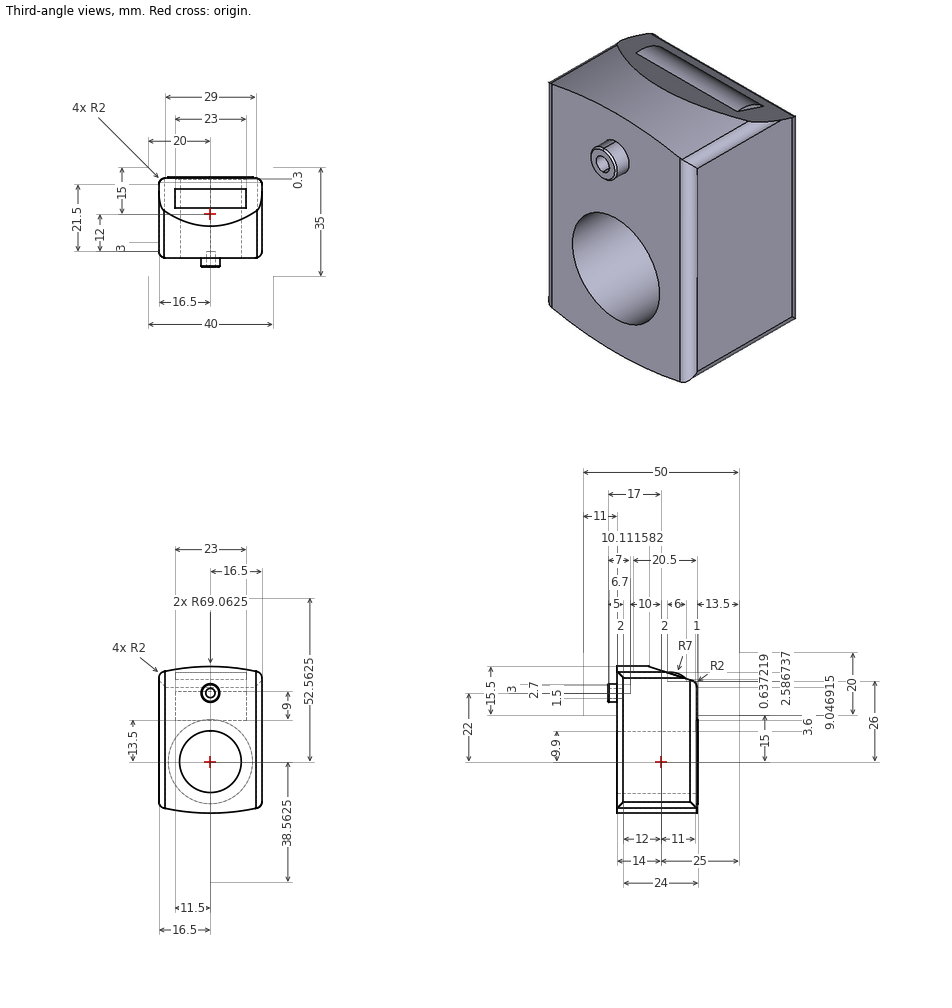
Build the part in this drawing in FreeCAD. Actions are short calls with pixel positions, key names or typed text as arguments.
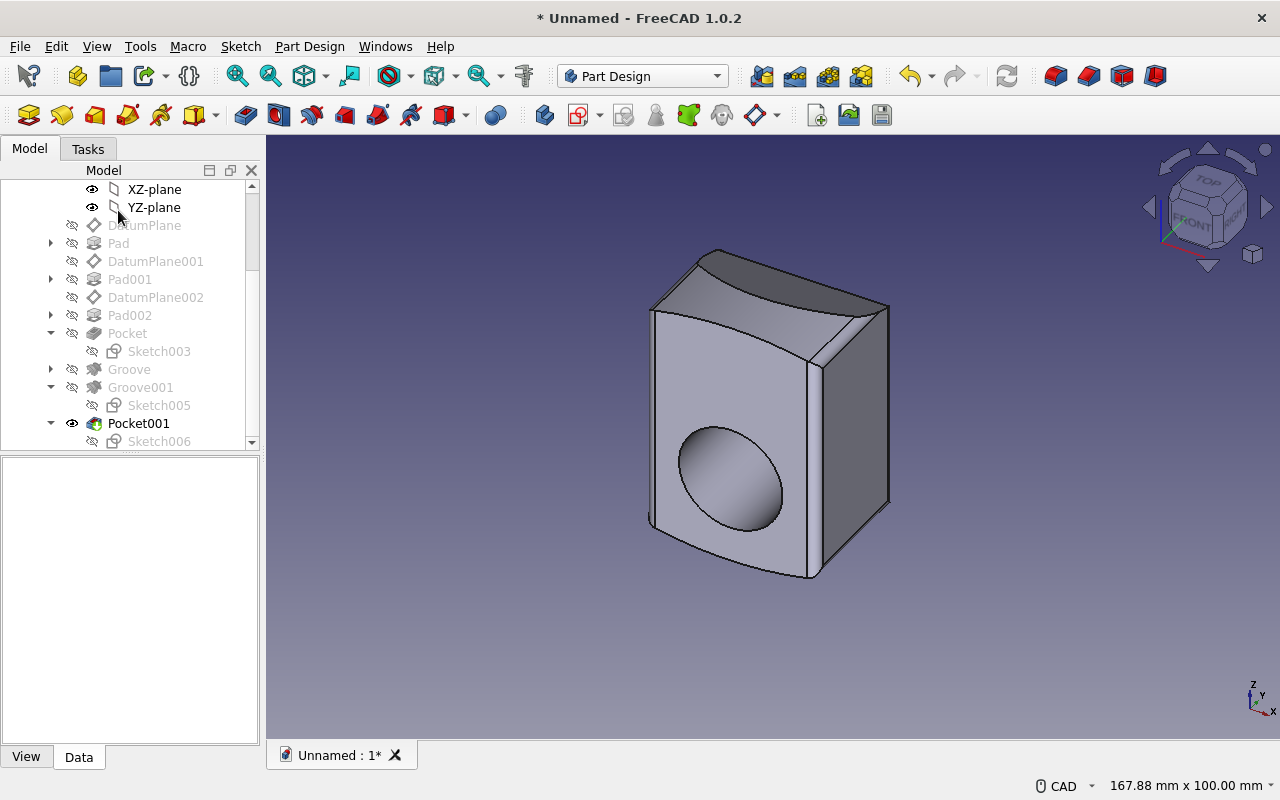
click(578, 116)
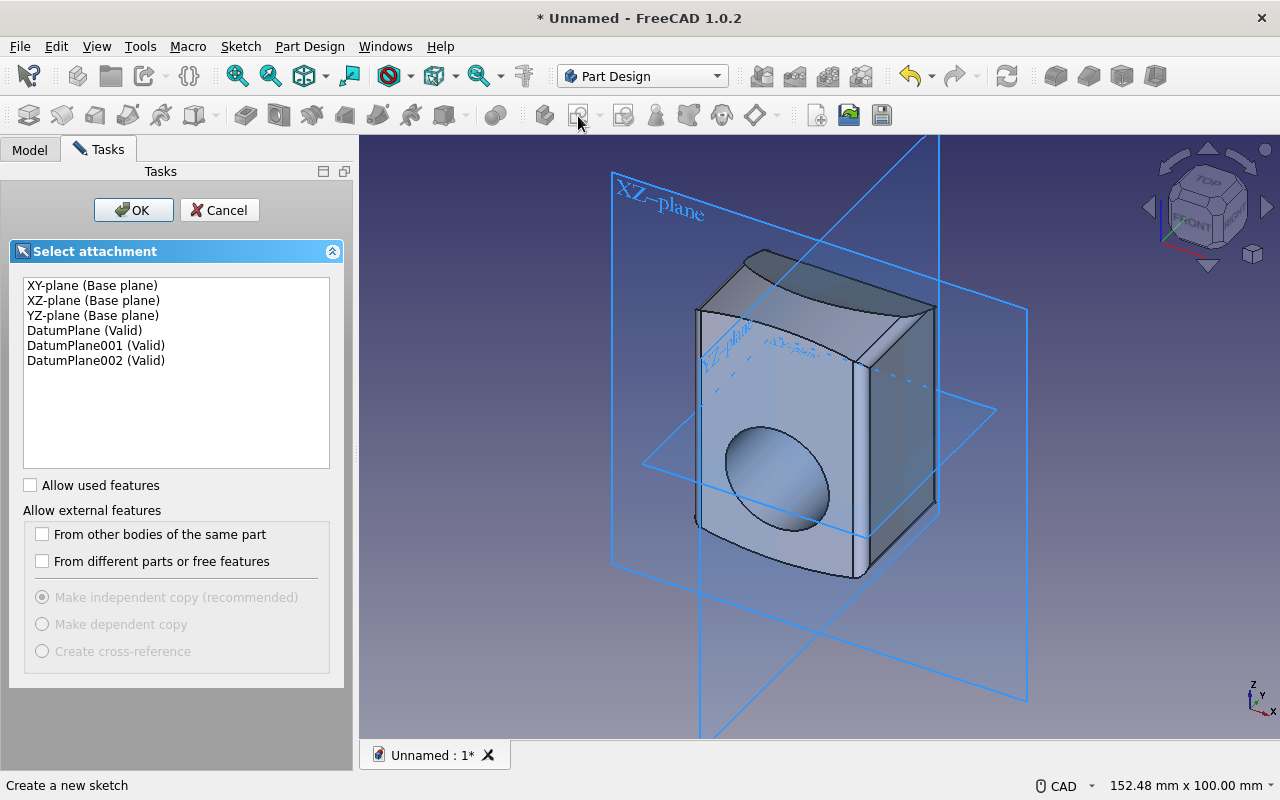
click(84, 316)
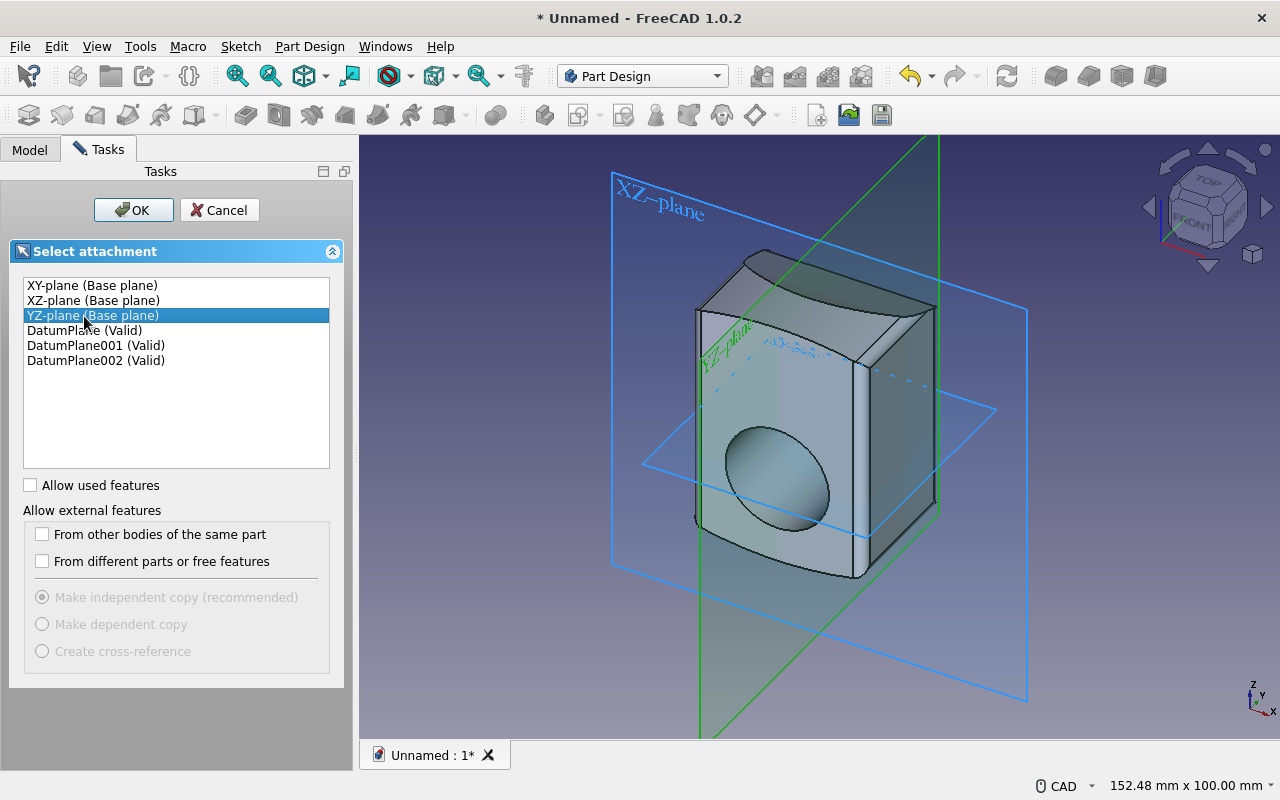
click(134, 210)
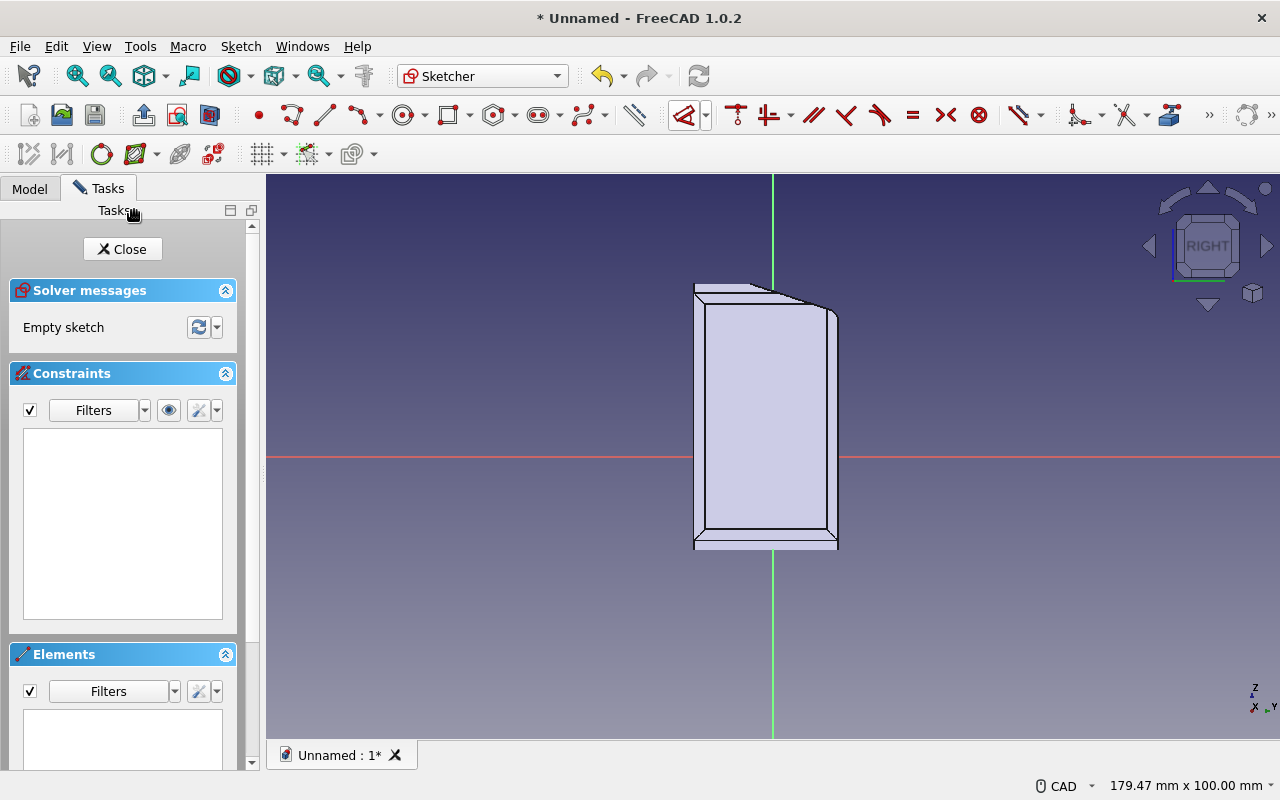
click(210, 116)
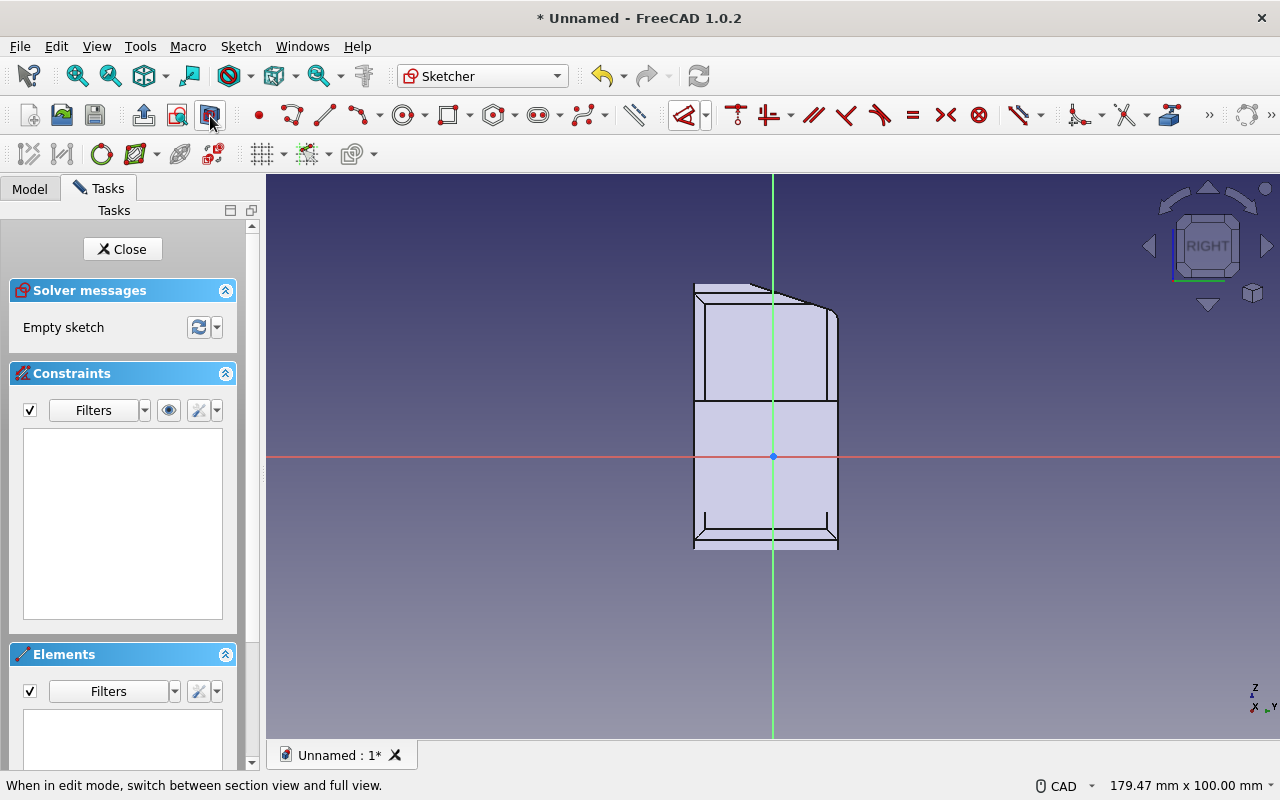
scroll(847, 386, up, 14)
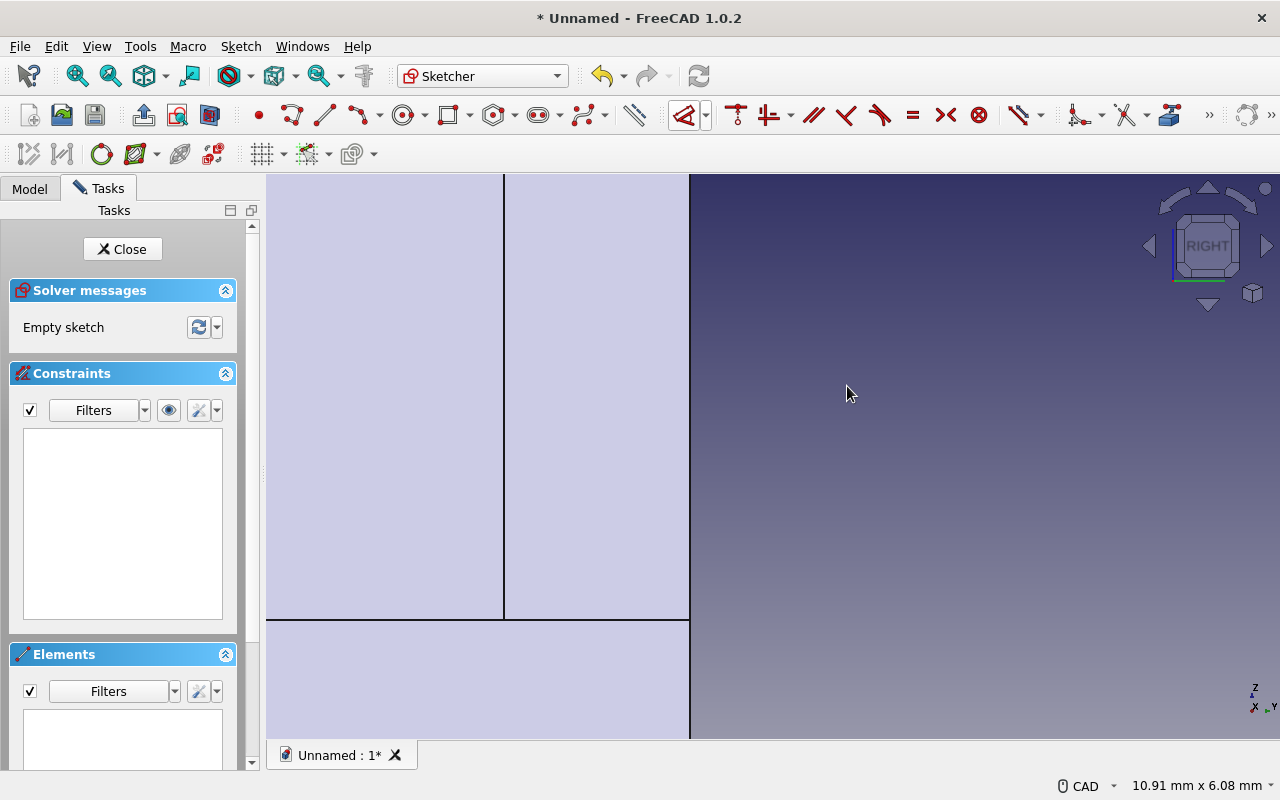
click(448, 116)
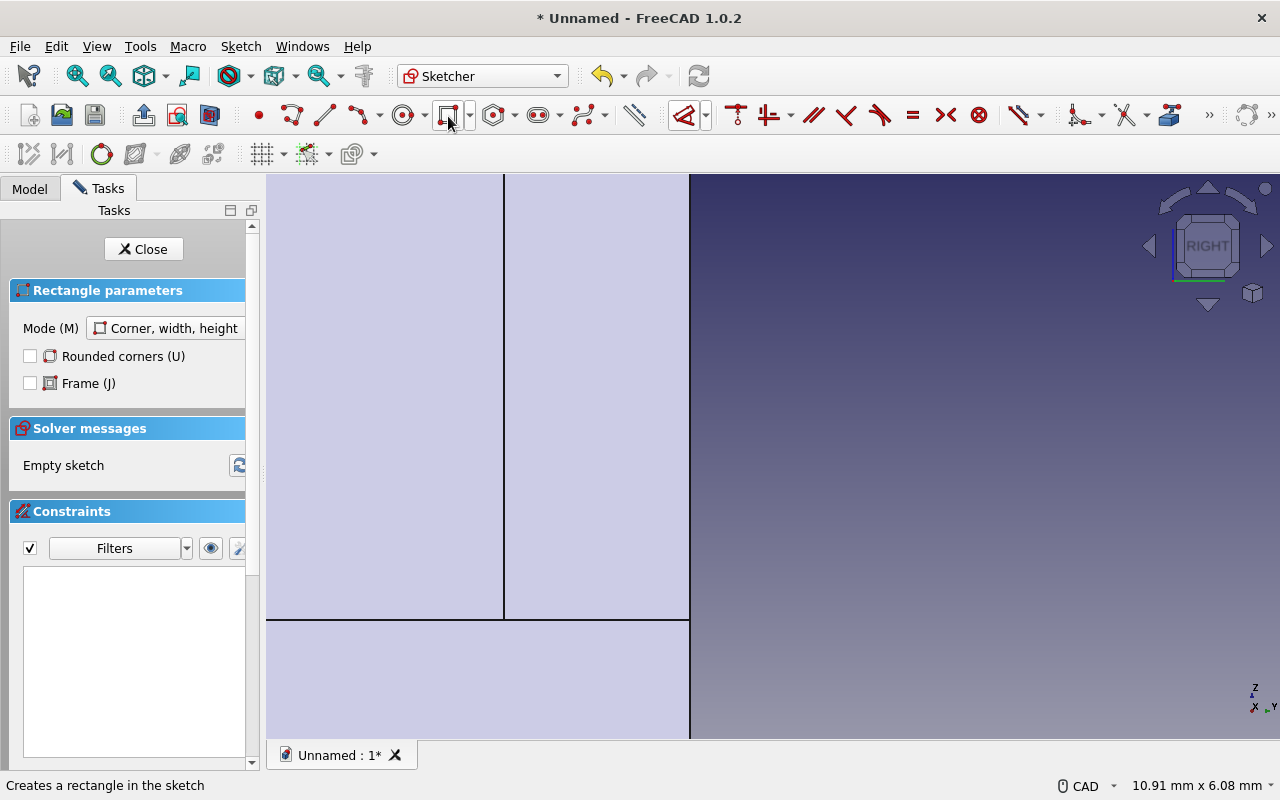
click(643, 285)
move(736, 620)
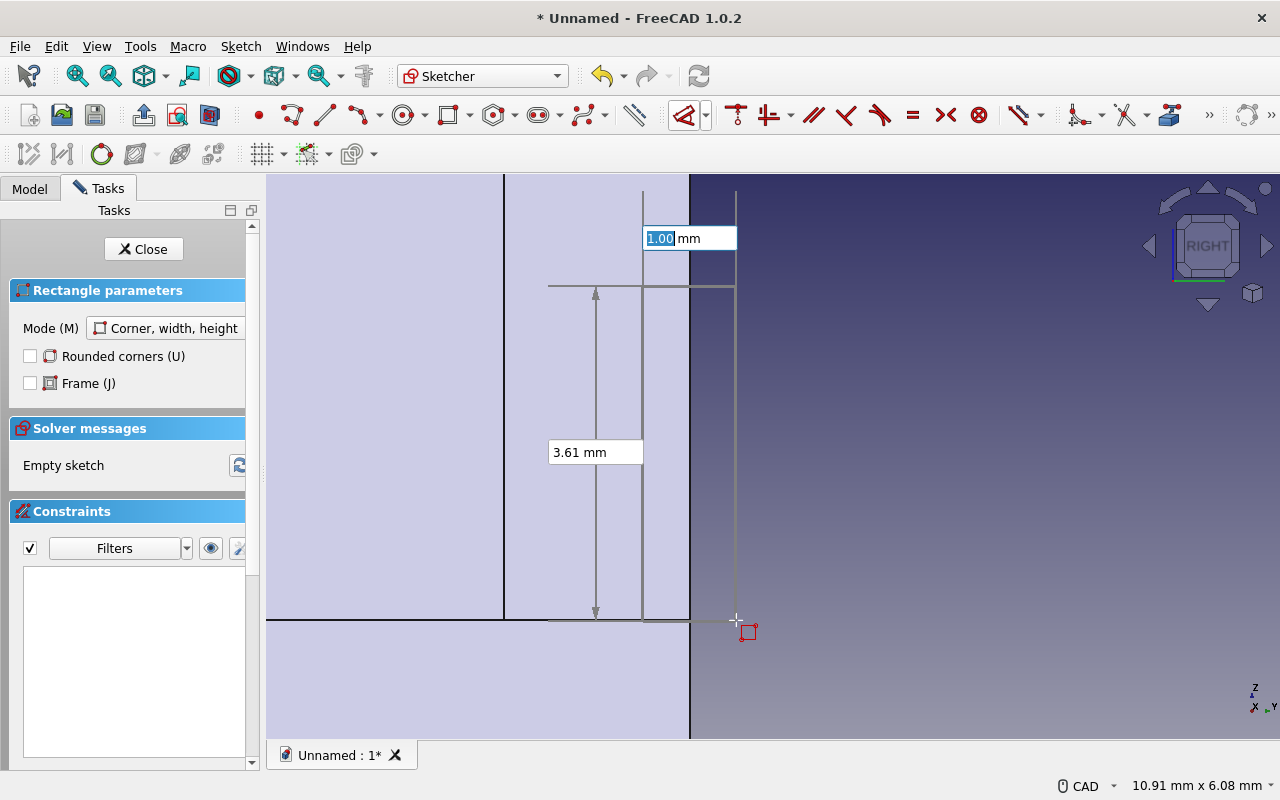
text(1)
key(Tab)
text(3.6)
key(Return)
key(Escape)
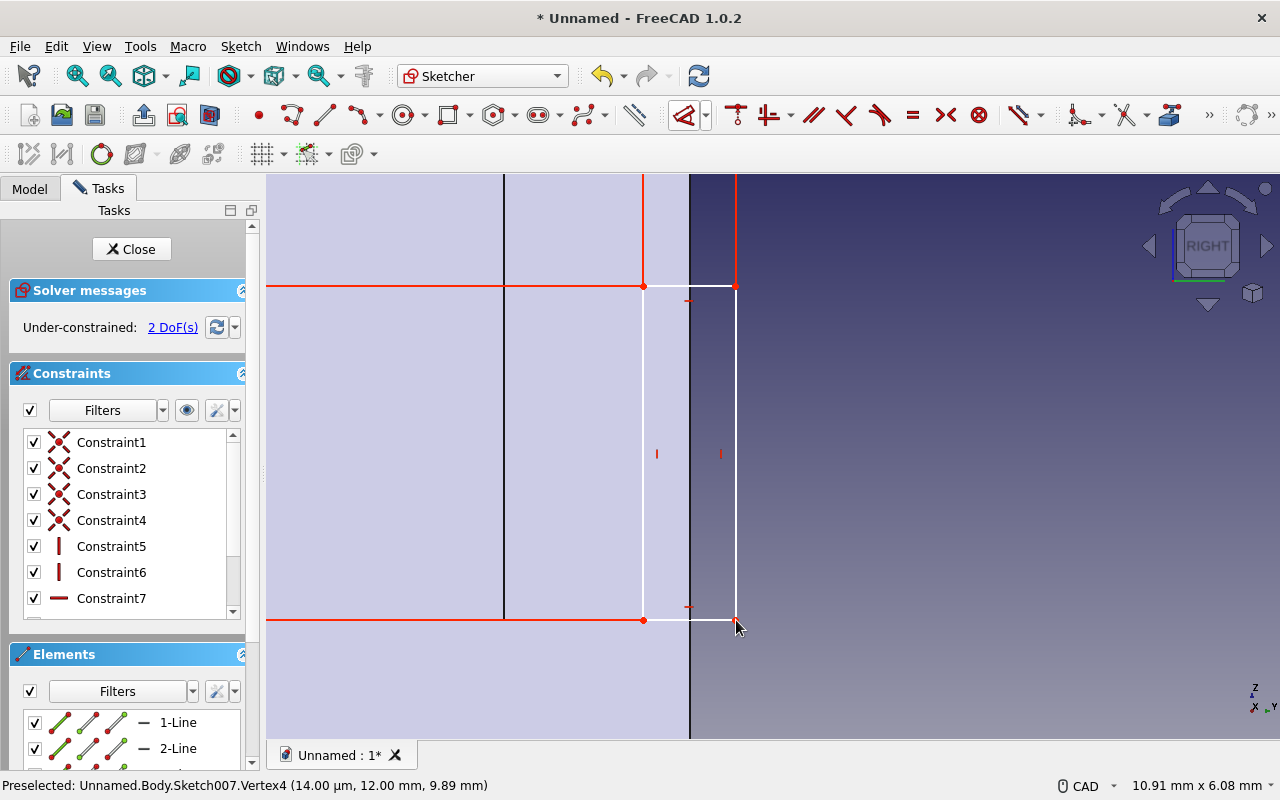
click(643, 286)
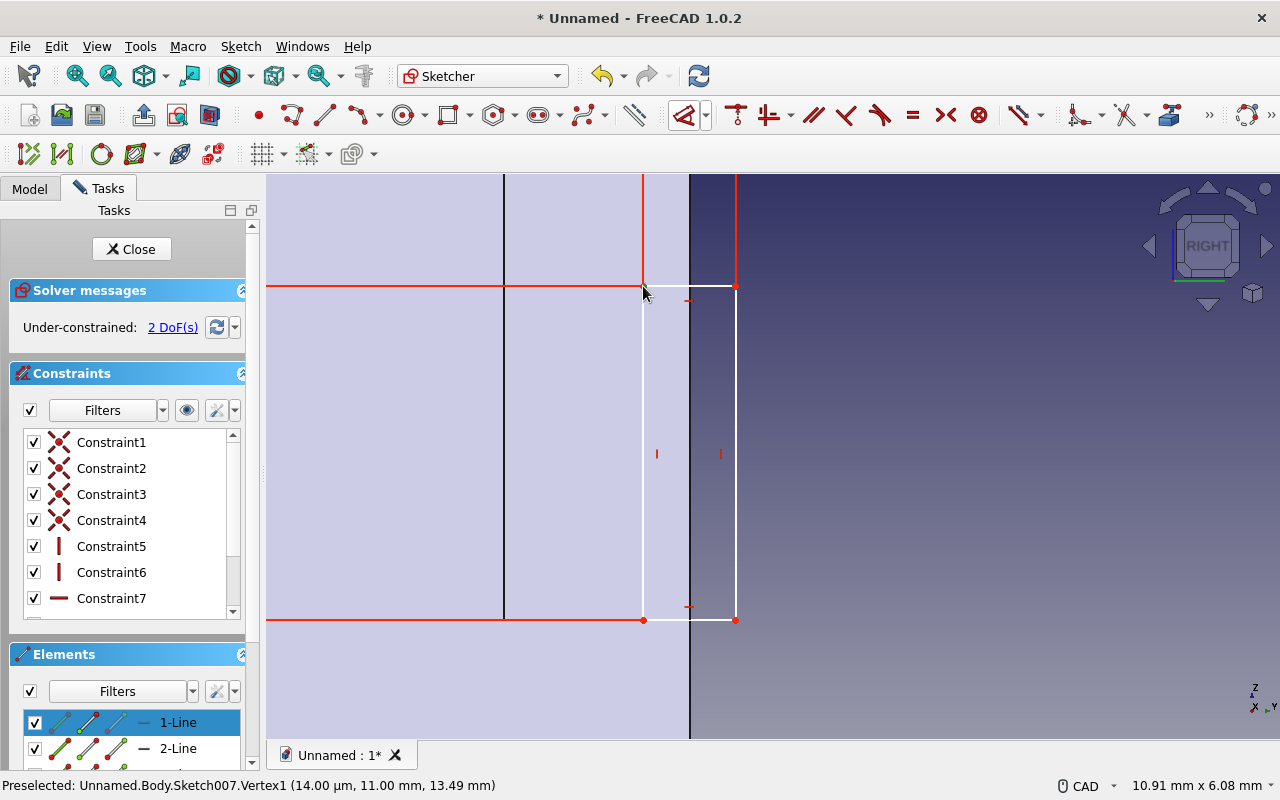
click(706, 116)